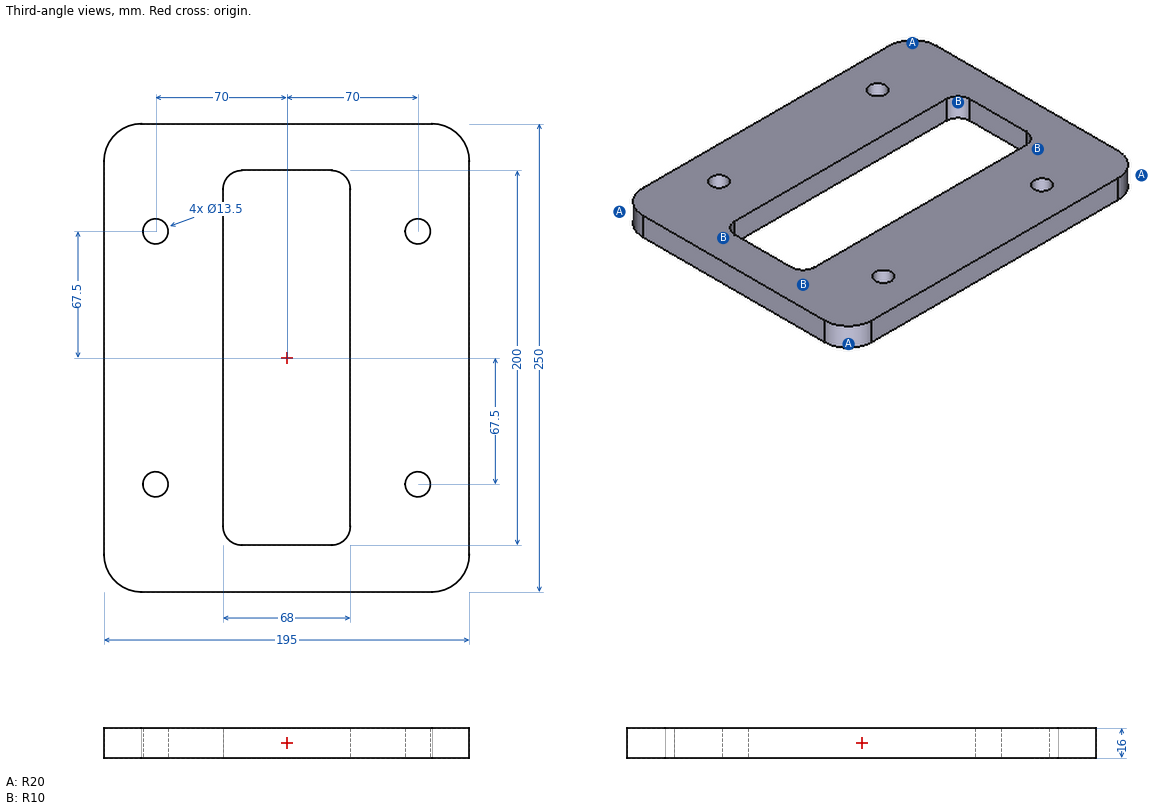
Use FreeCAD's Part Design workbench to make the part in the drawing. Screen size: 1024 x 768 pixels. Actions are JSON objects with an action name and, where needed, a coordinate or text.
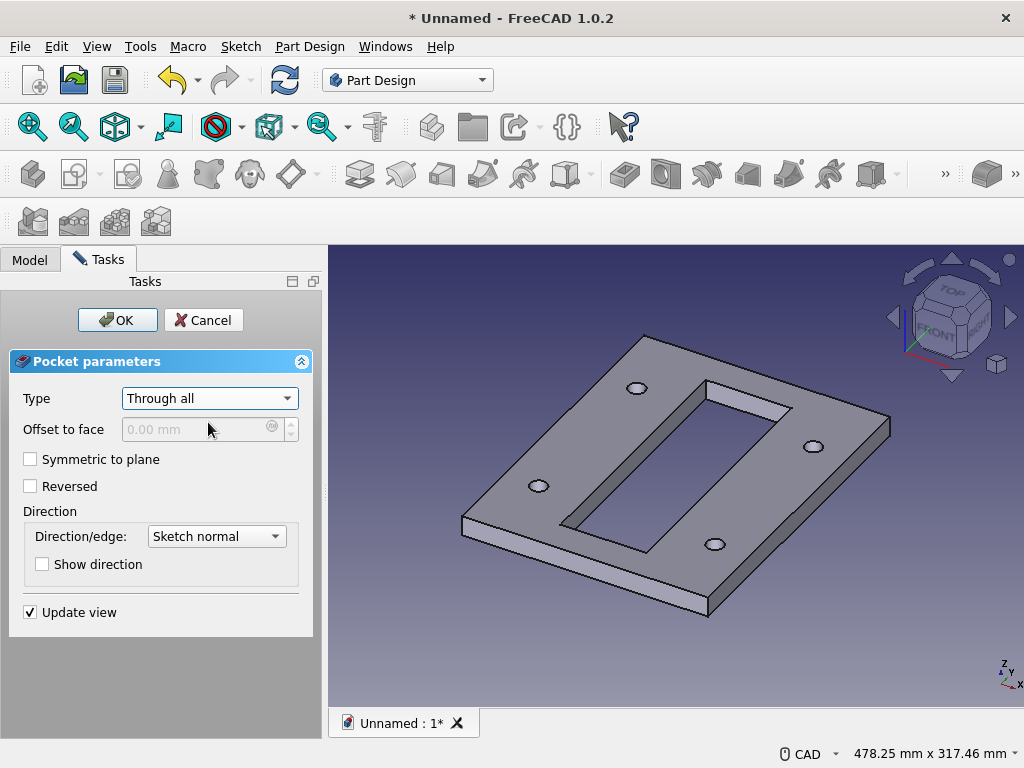
{"action": "left_click", "coordinate": [118, 320]}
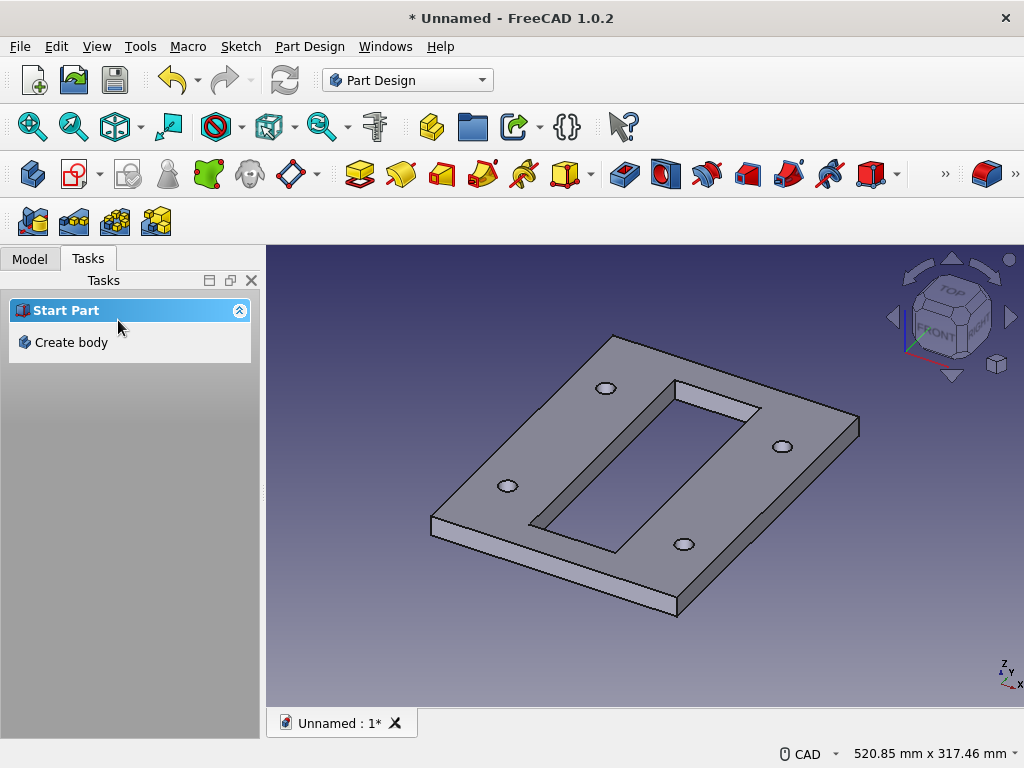
{"action": "left_click", "coordinate": [677, 606]}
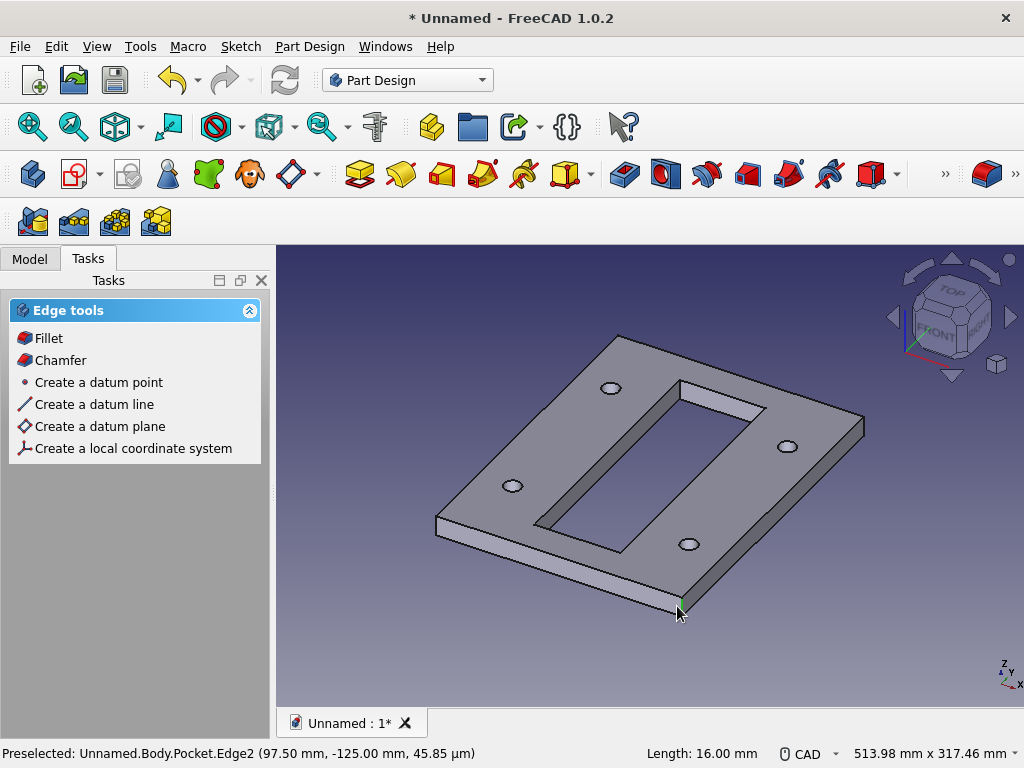
{"action": "key", "text": "0"}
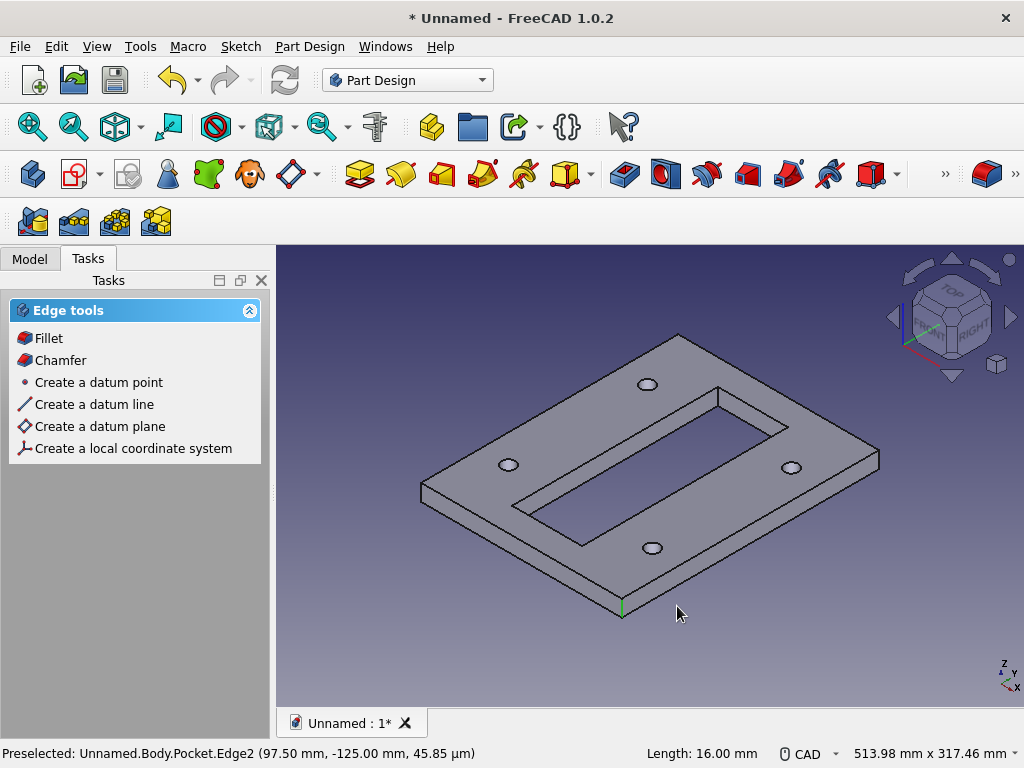
{"action": "key", "text": "2"}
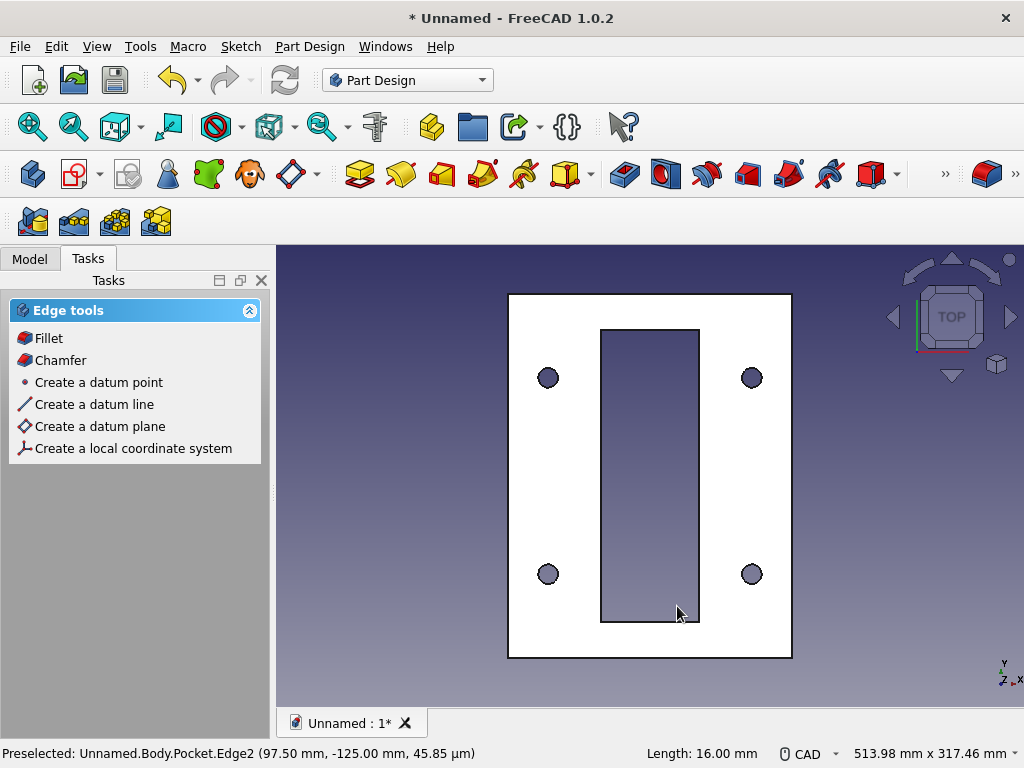
{"action": "key", "text": "1"}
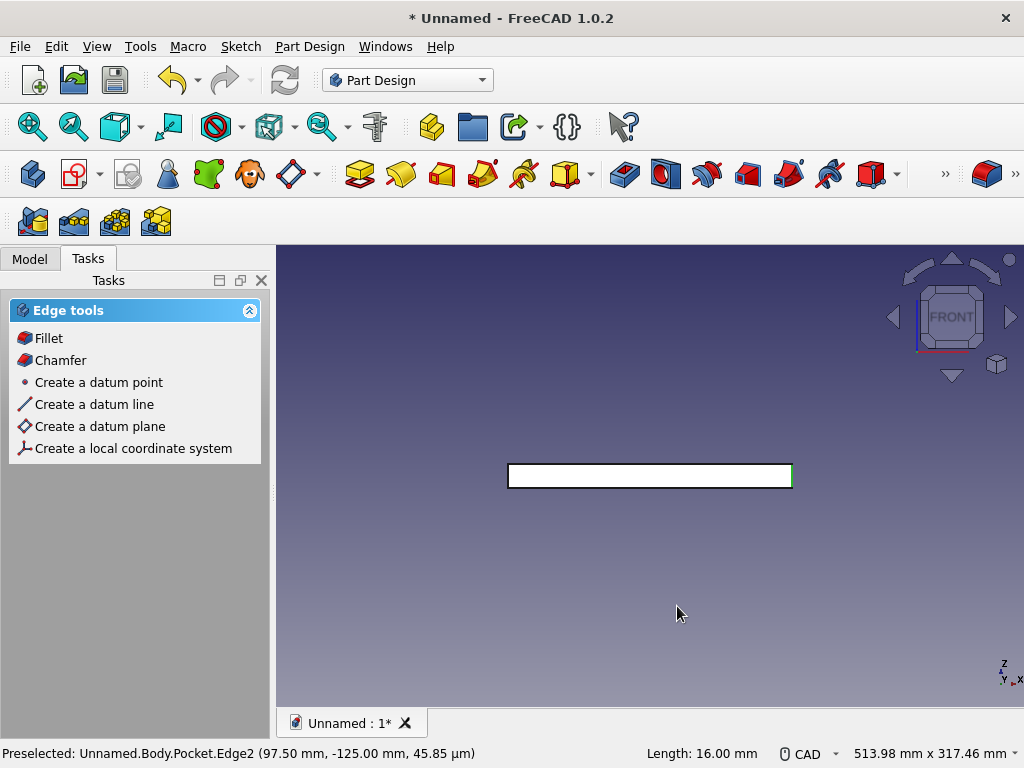
{"action": "left_click", "coordinate": [33, 128]}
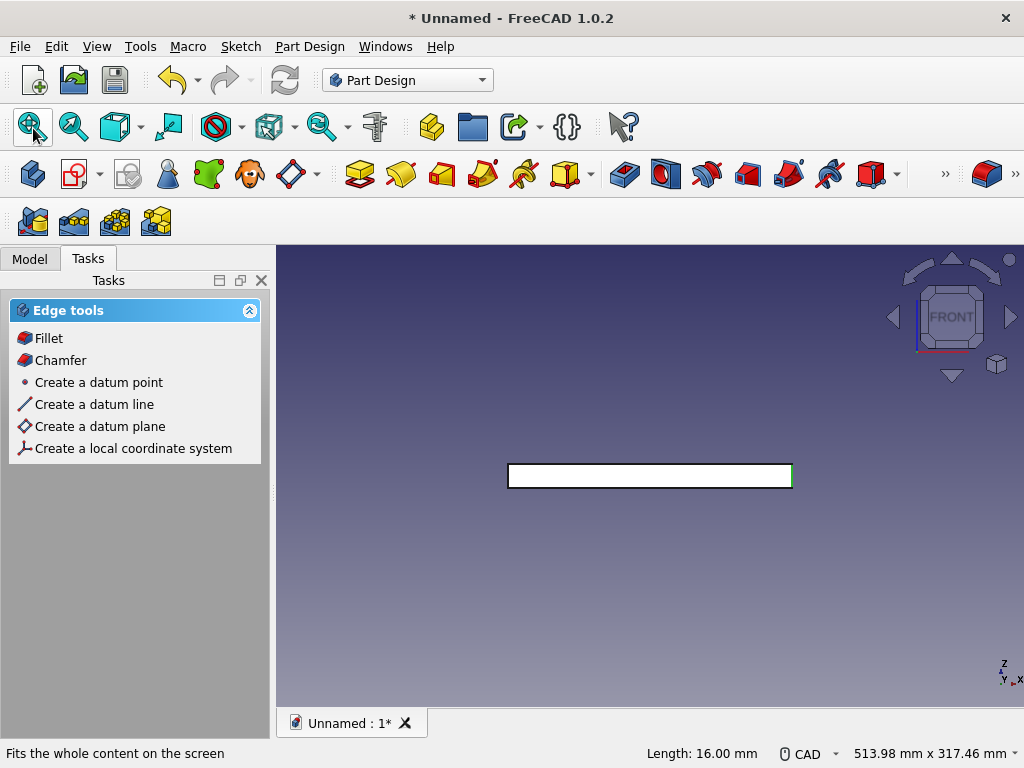
{"action": "left_click", "coordinate": [508, 475], "text": "ctrl"}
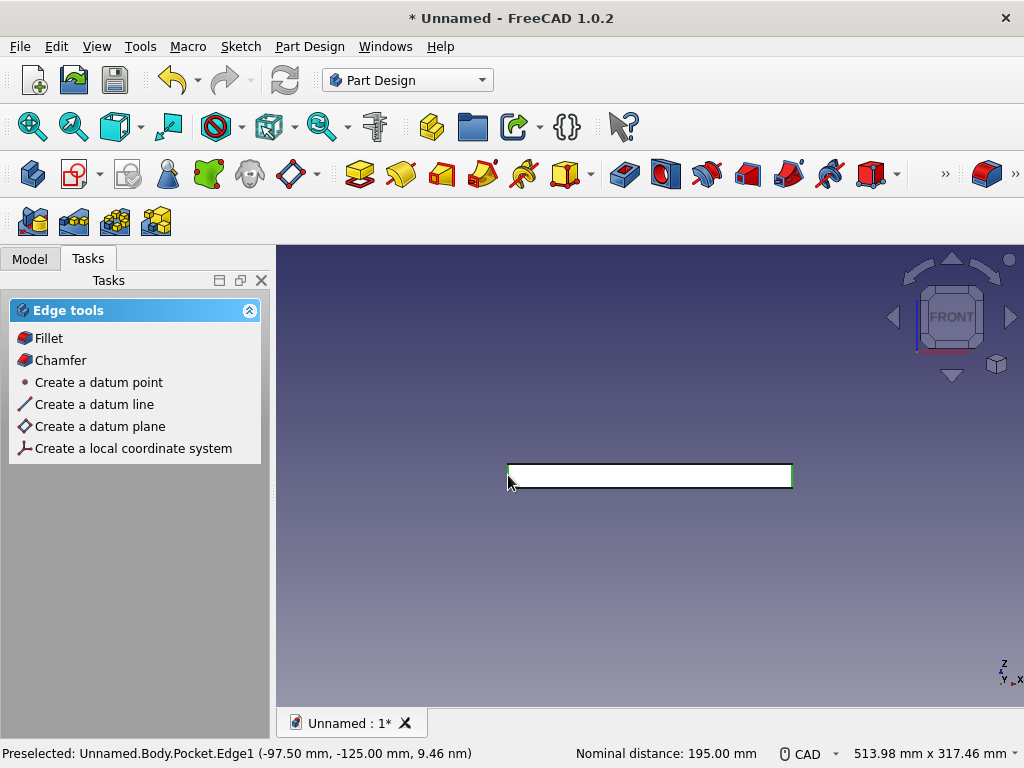
{"action": "key", "text": "3"}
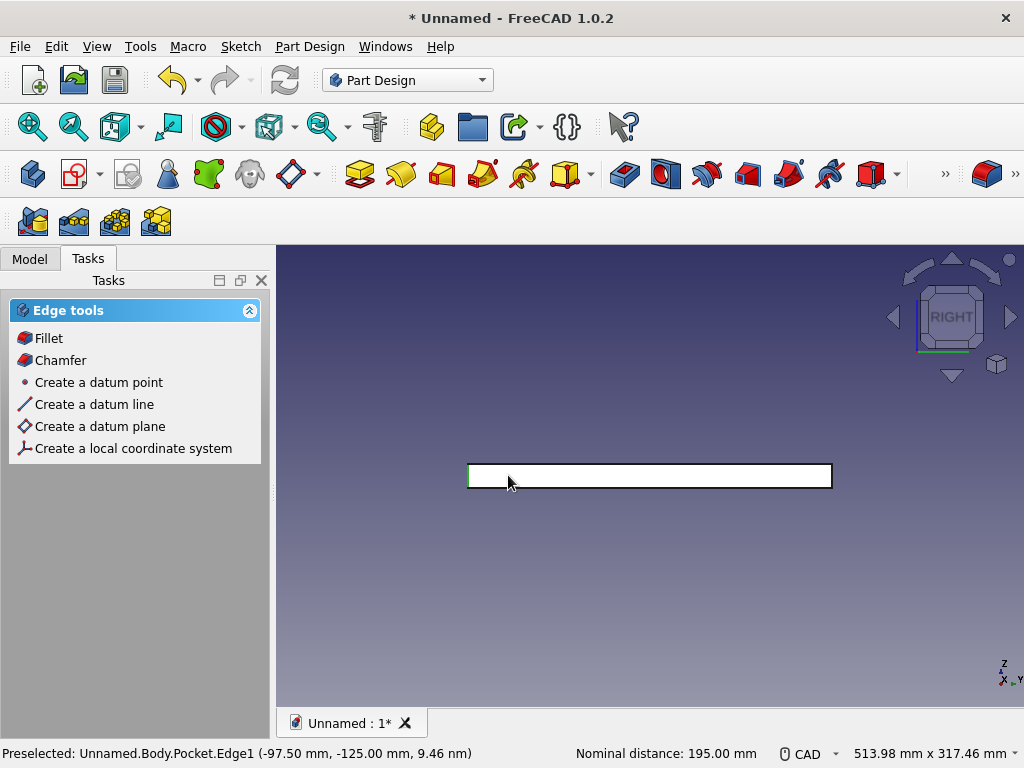
{"action": "left_click", "coordinate": [832, 475], "text": "ctrl"}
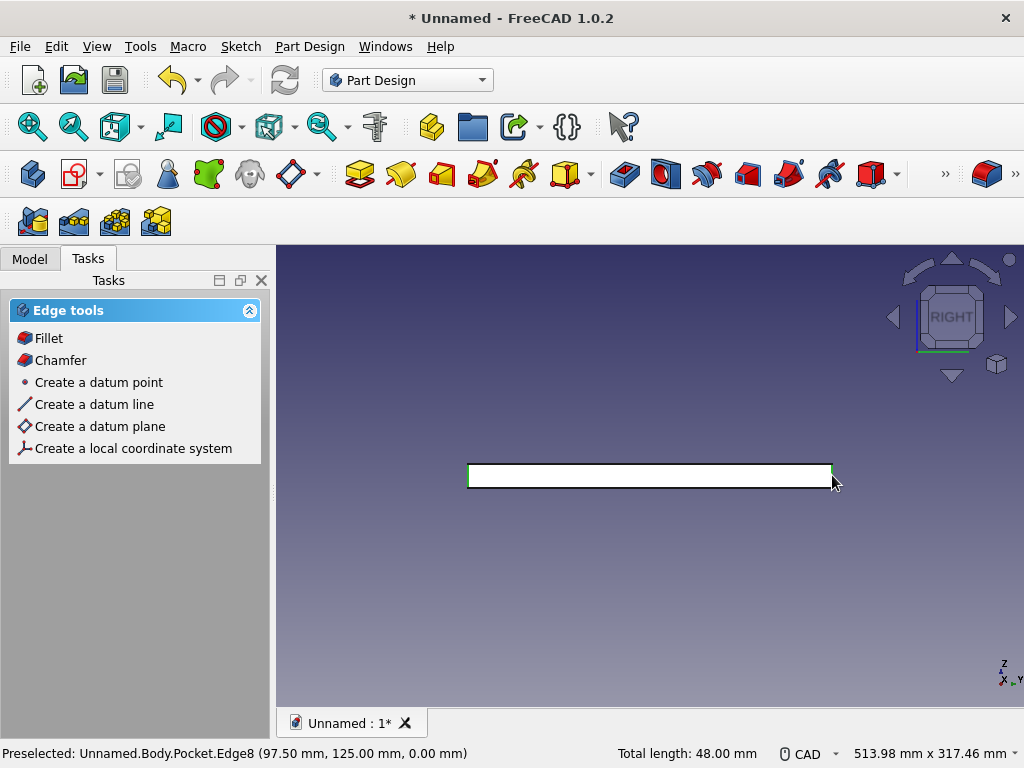
{"action": "key", "text": "5"}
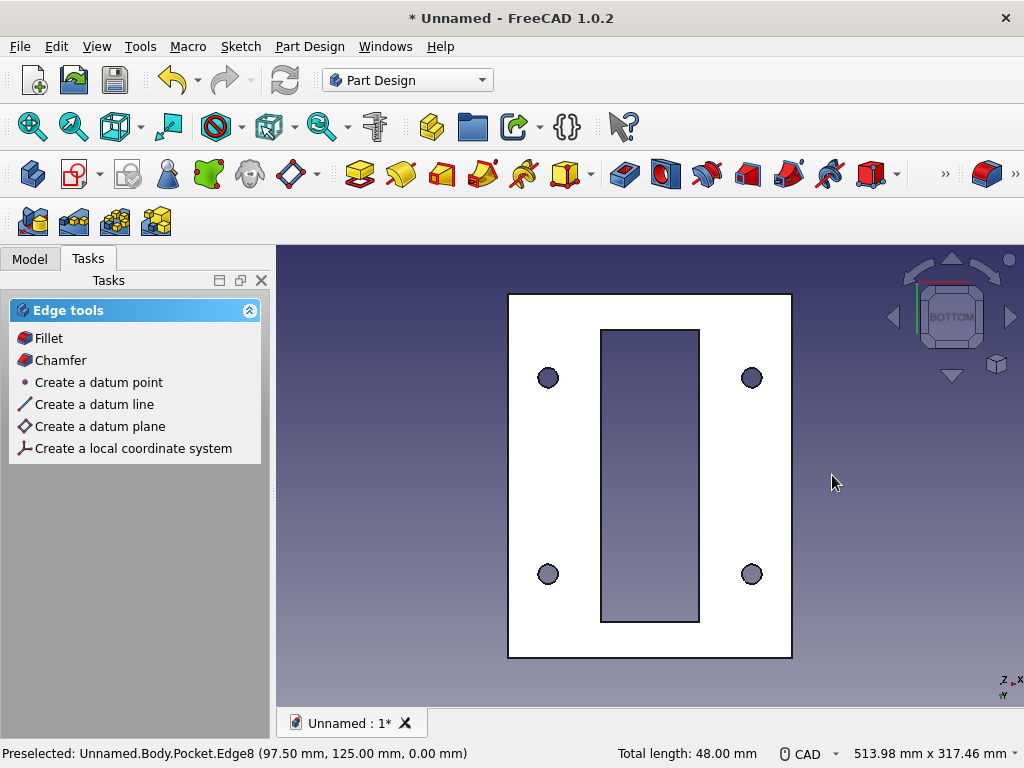
{"action": "key", "text": "4"}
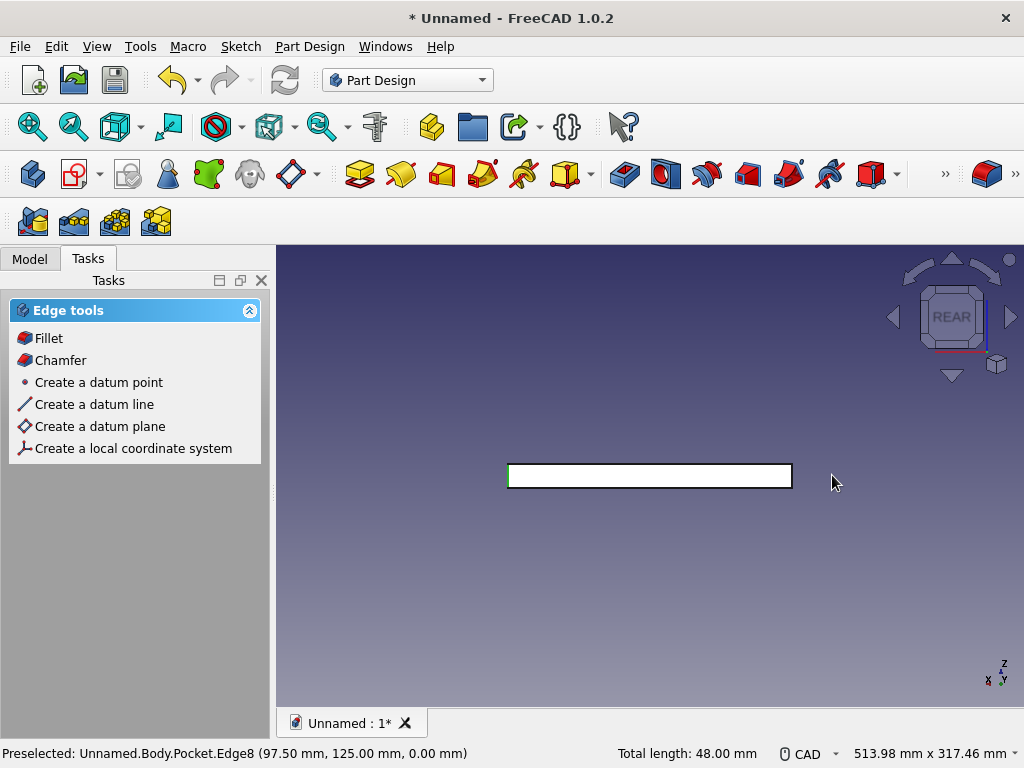
{"action": "left_click", "coordinate": [33, 128]}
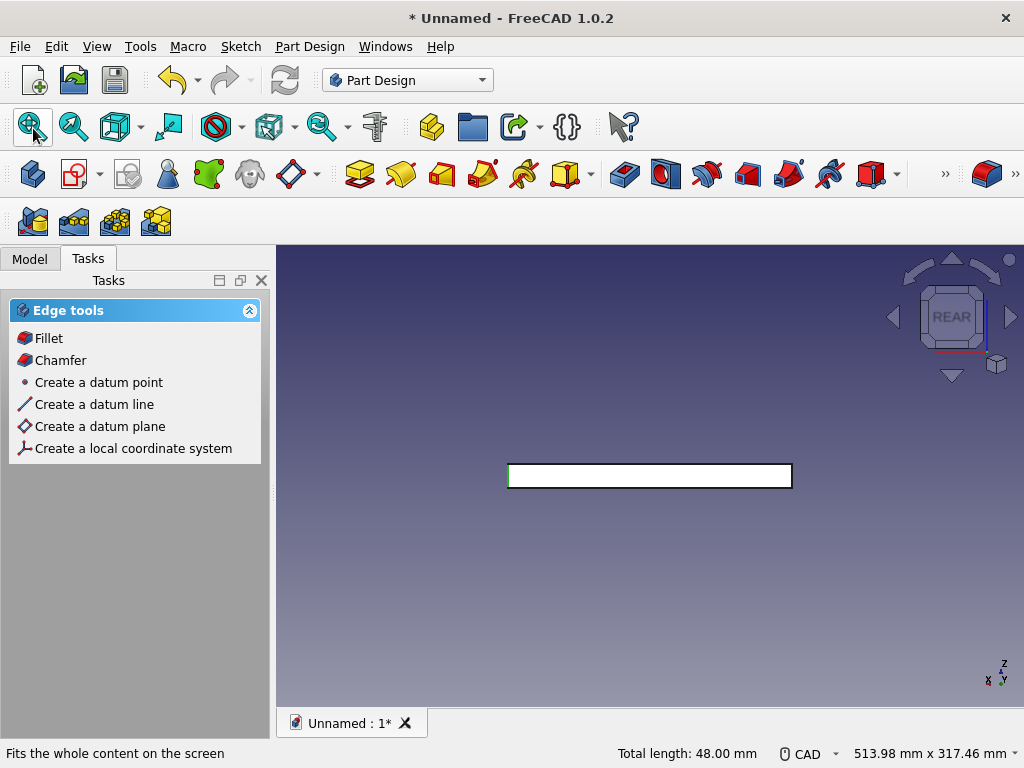
{"action": "left_click", "coordinate": [792, 475], "text": "ctrl"}